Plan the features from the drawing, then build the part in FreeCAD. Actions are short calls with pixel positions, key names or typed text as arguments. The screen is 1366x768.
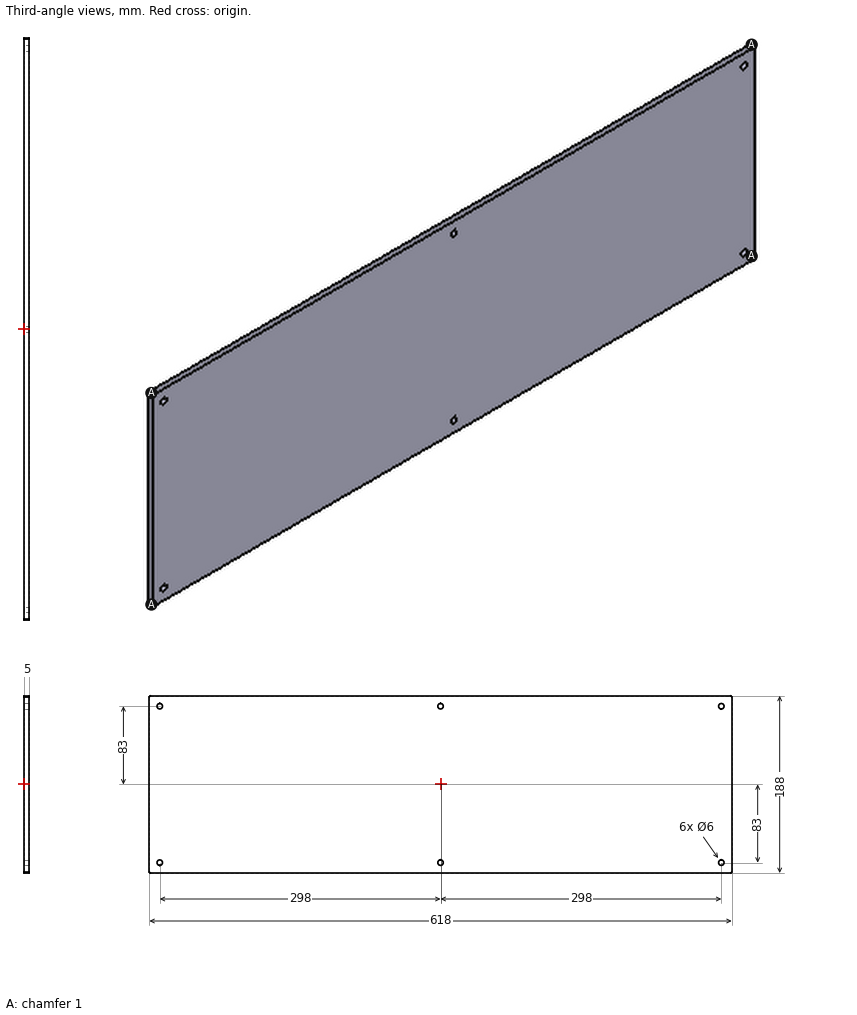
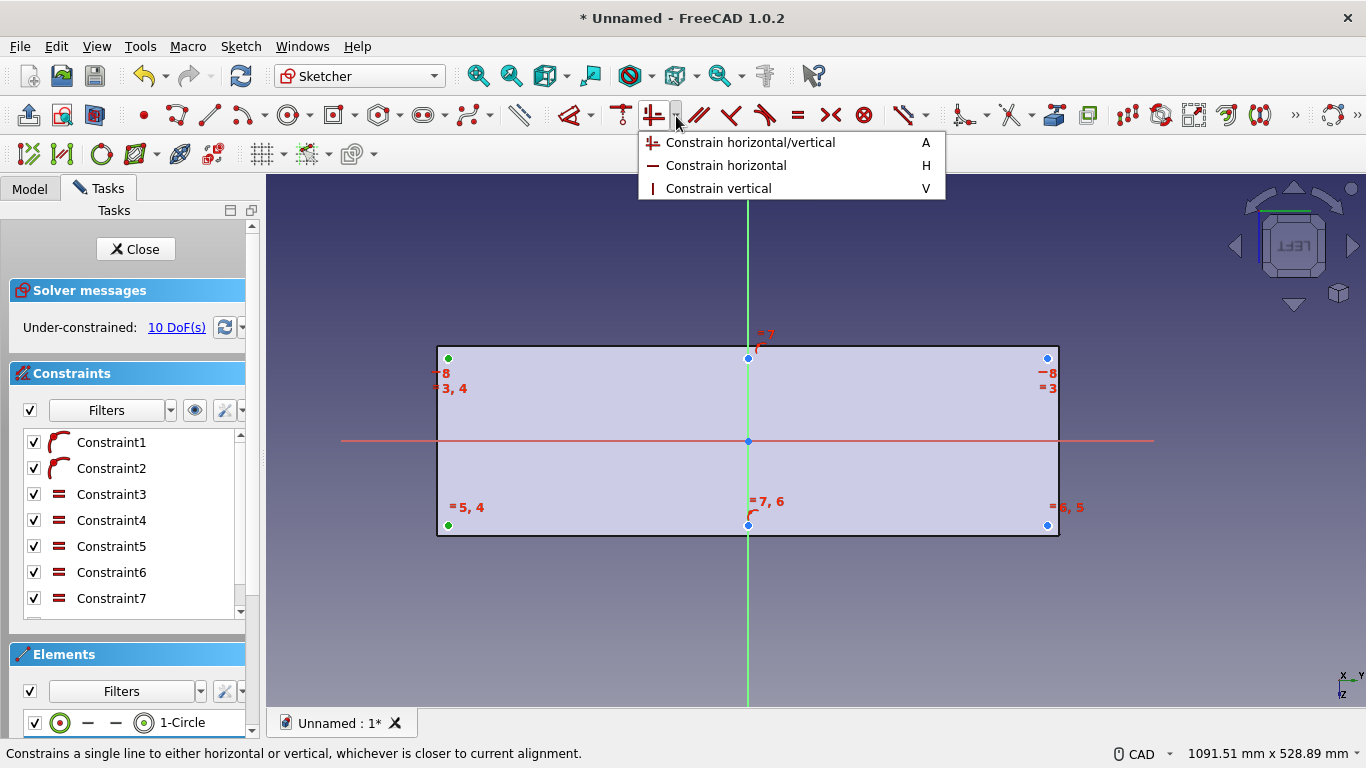
click(792, 188)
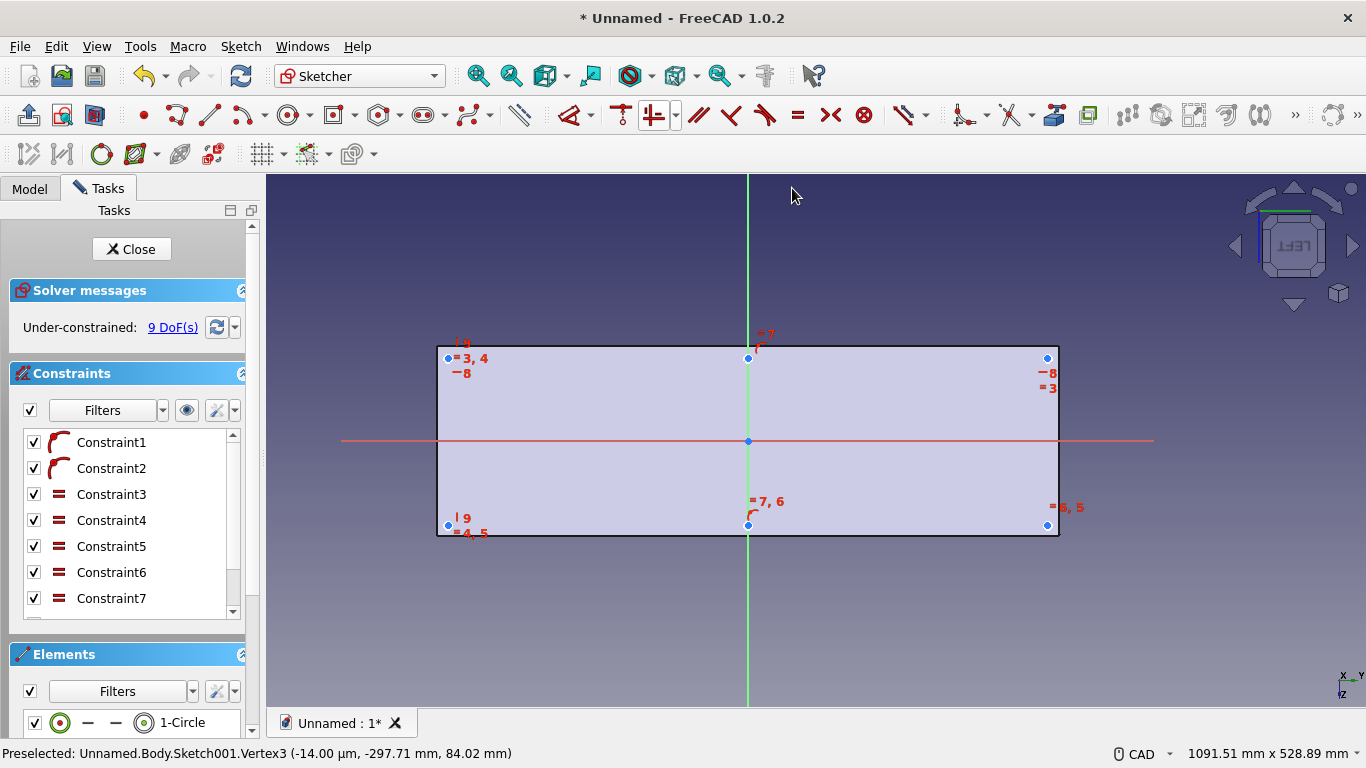
click(1048, 359)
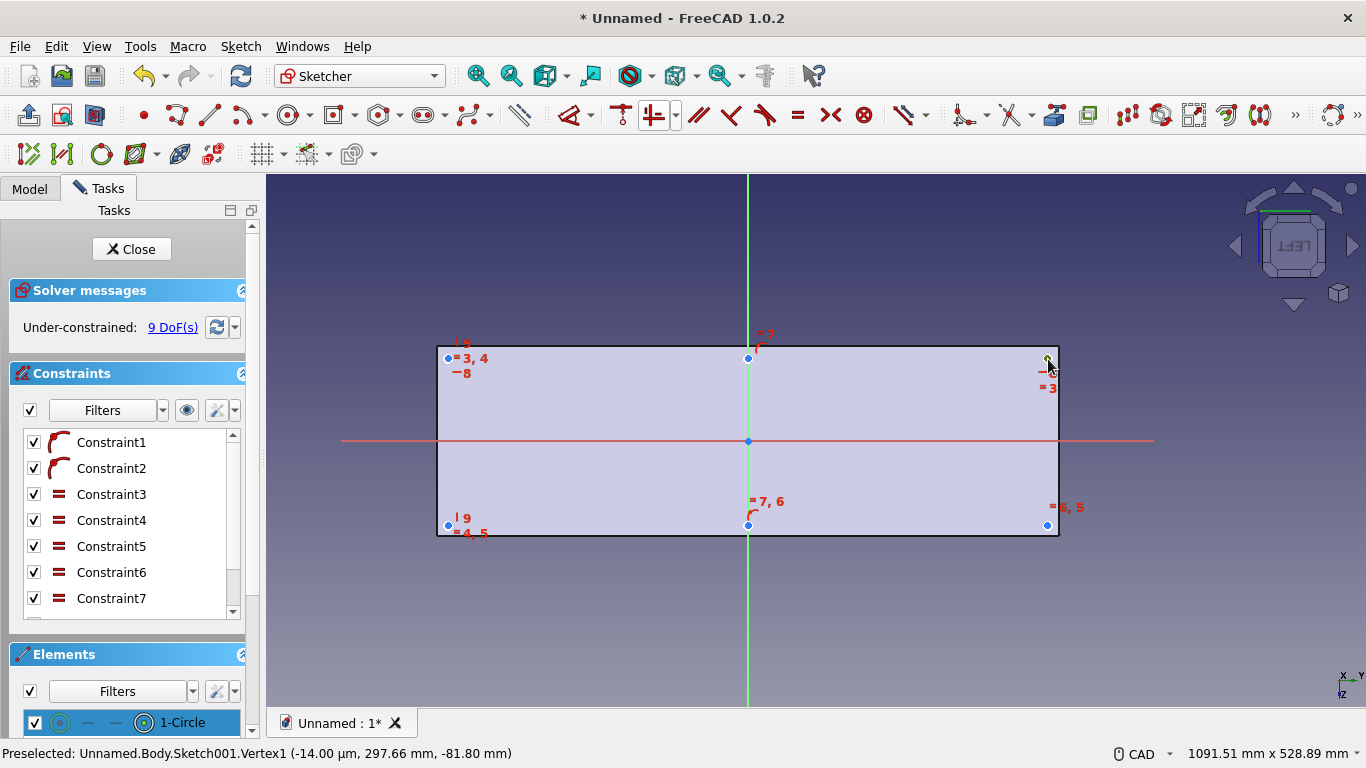
click(1048, 526)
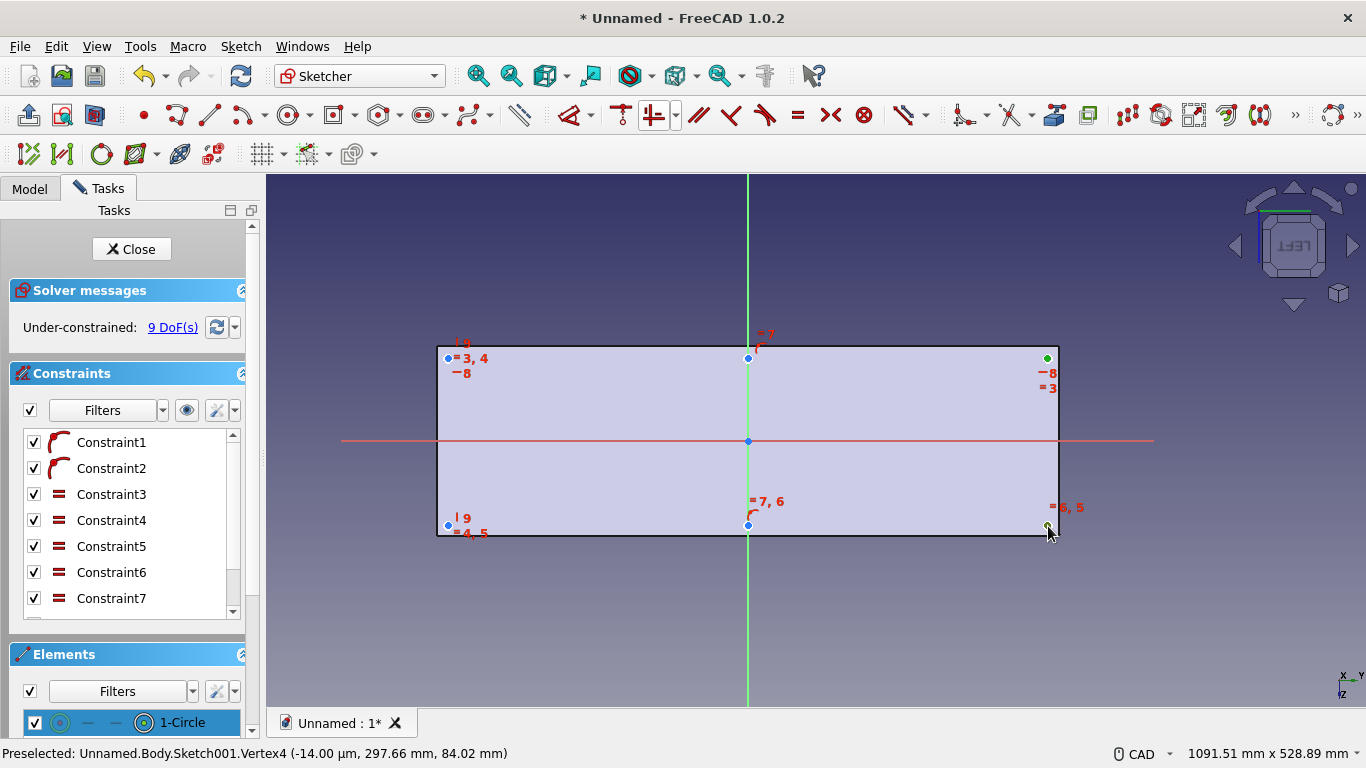
key(v)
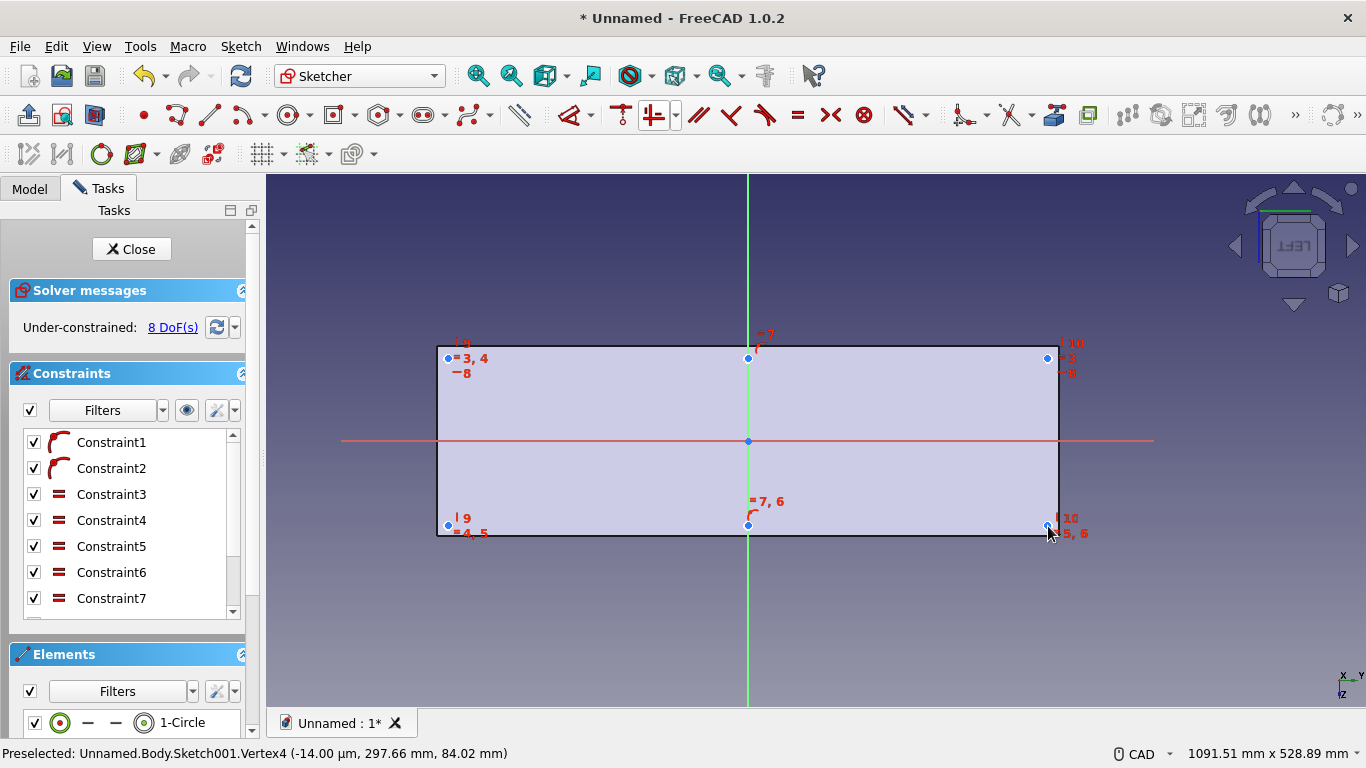
click(448, 526)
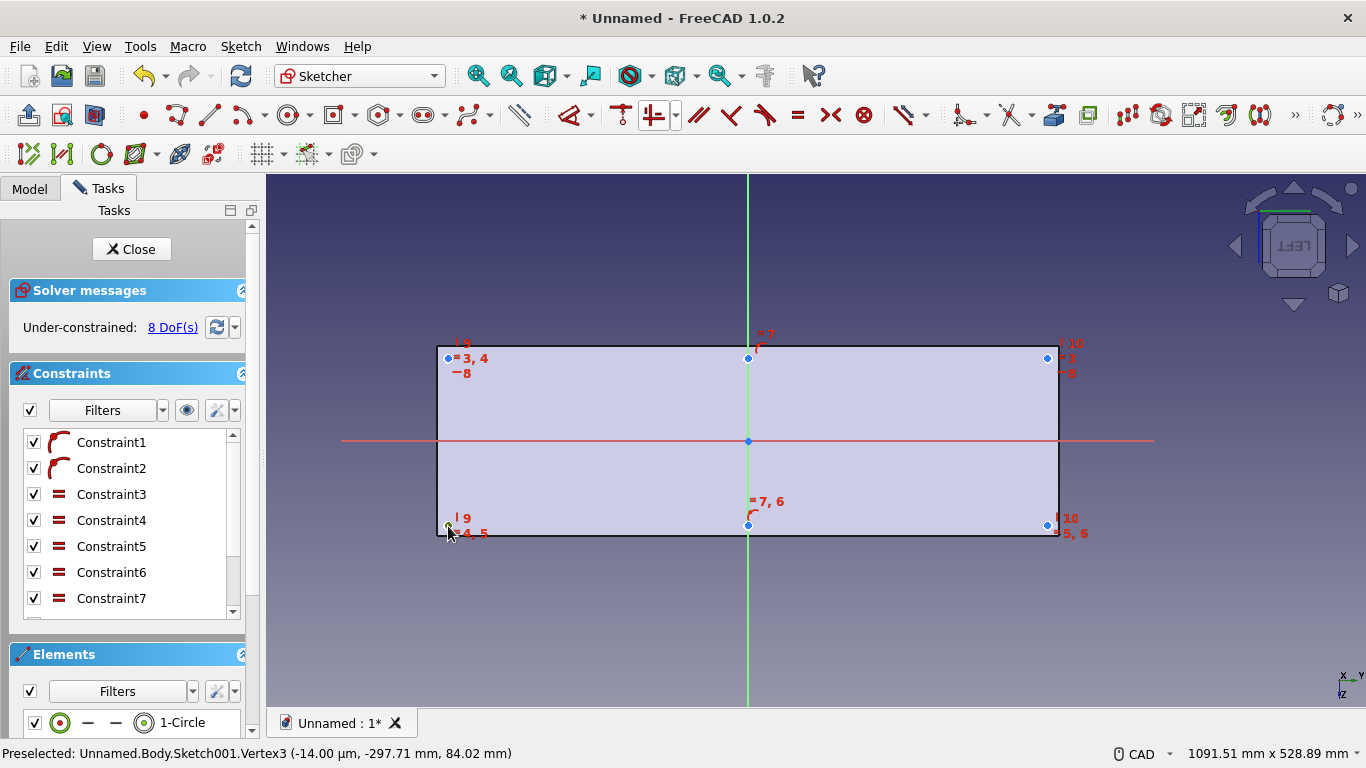
click(1048, 526)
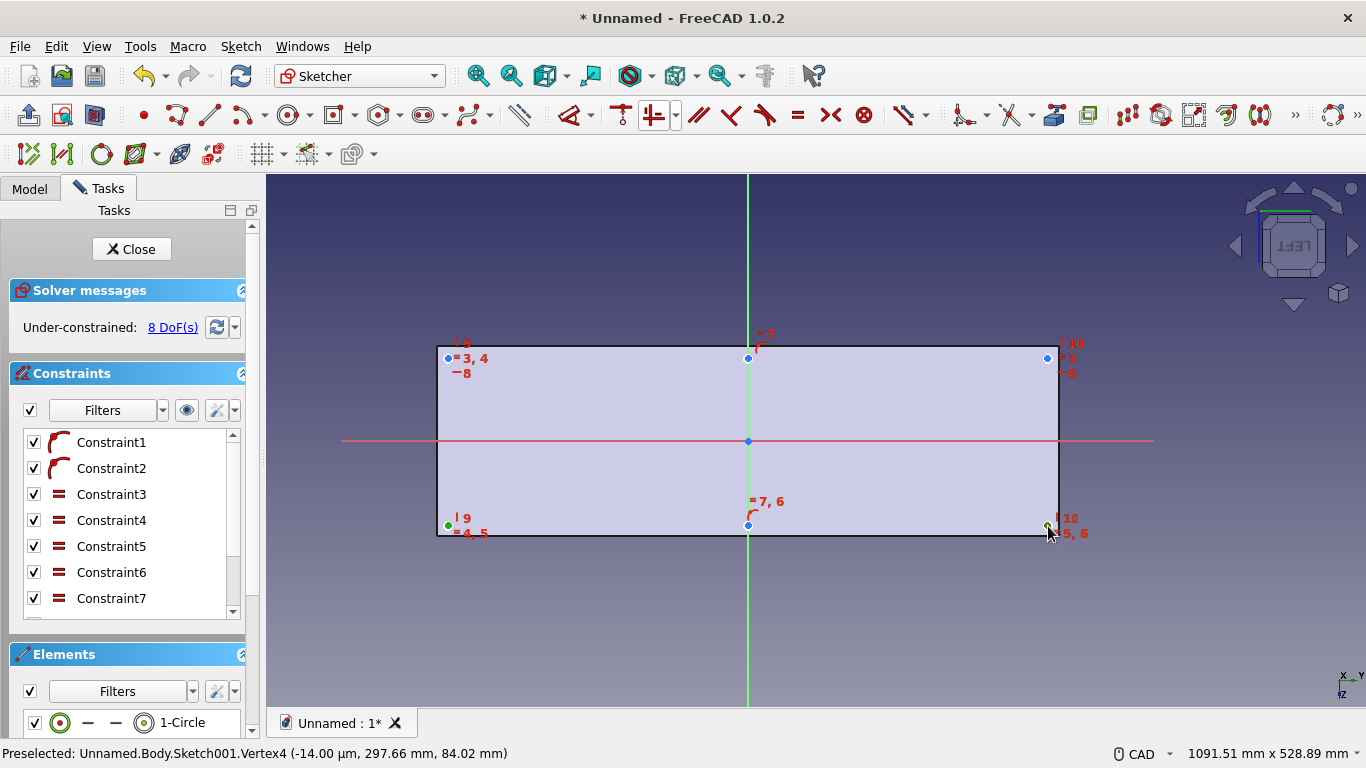
key(h)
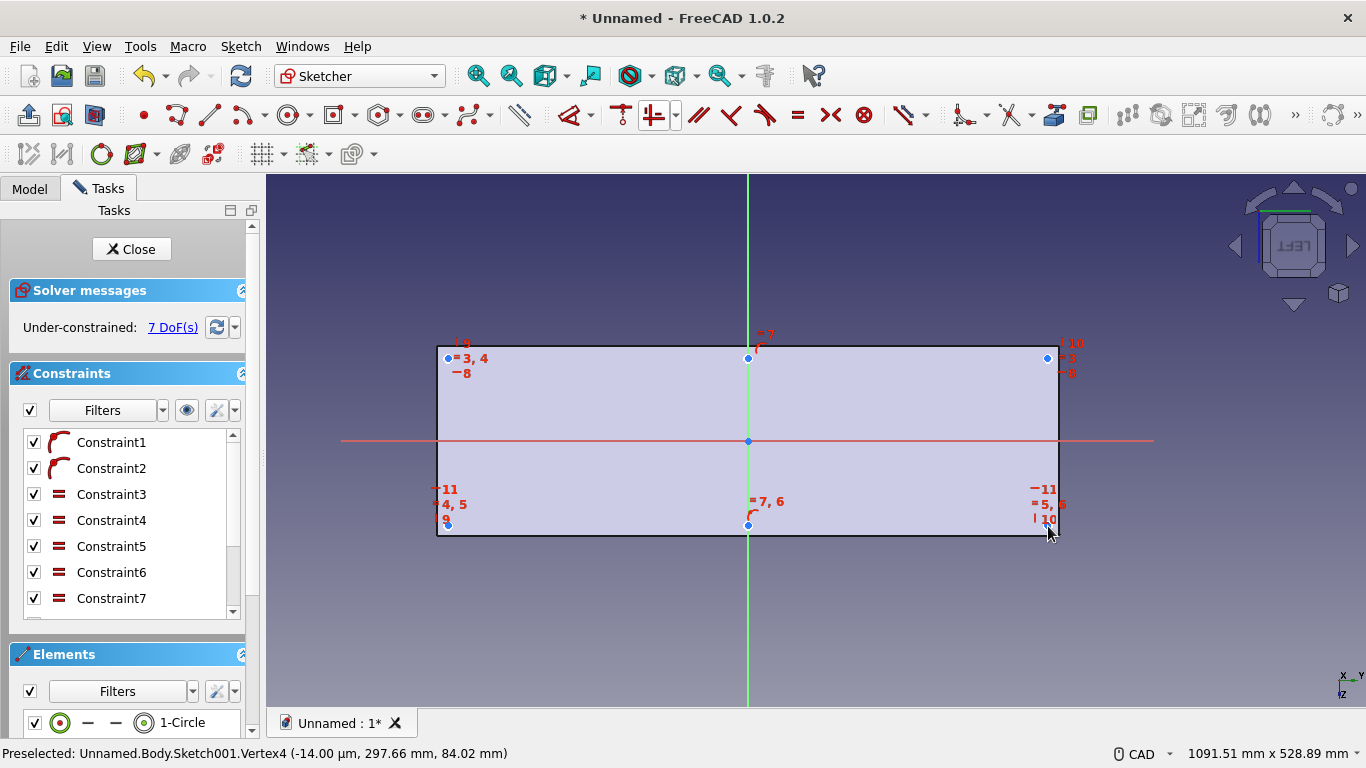
click(448, 526)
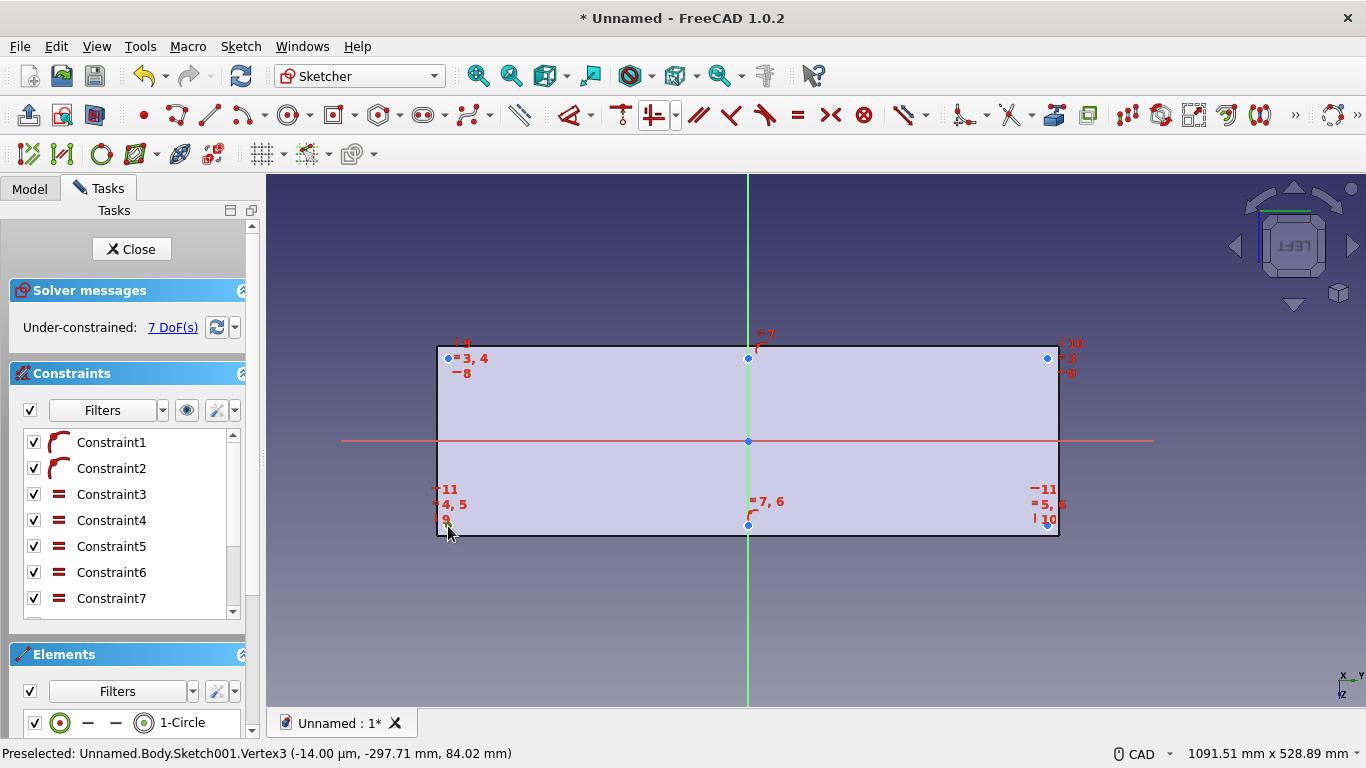
click(748, 526)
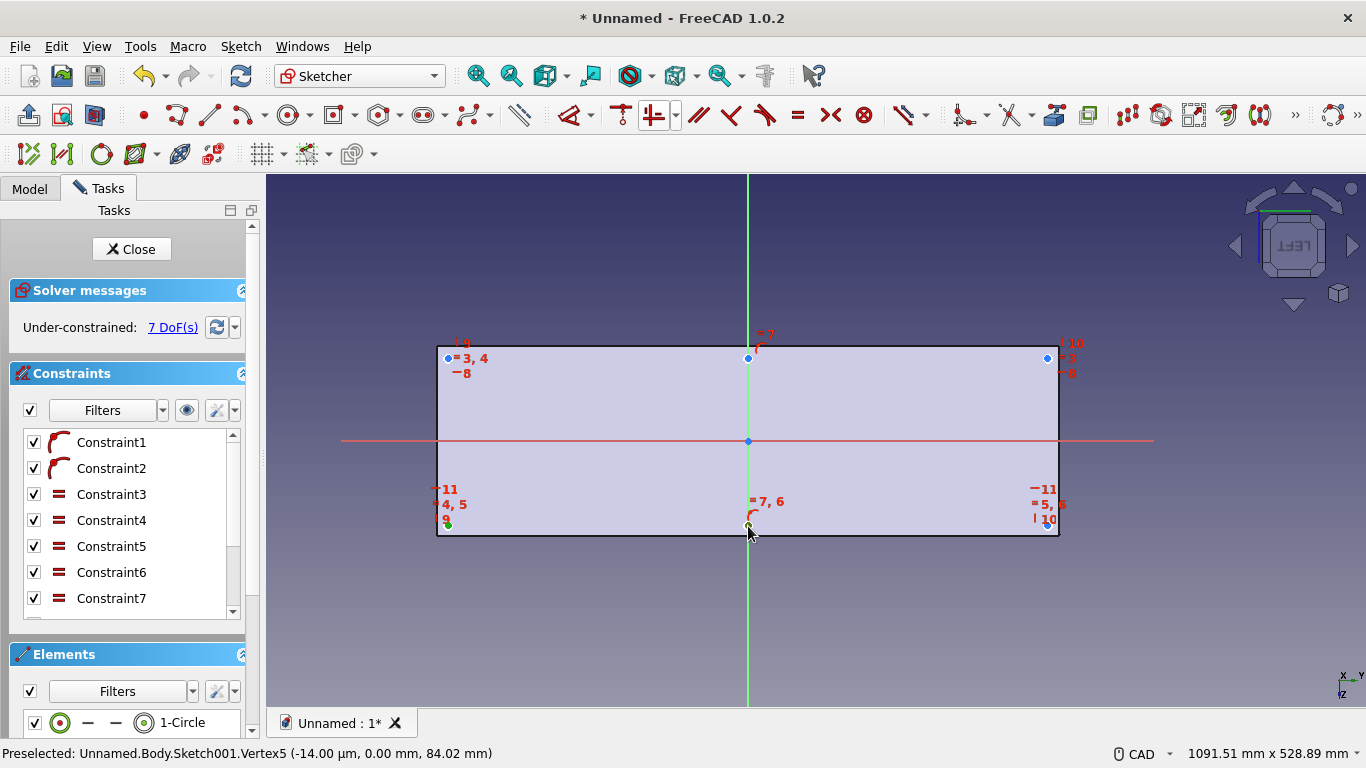
click(676, 116)